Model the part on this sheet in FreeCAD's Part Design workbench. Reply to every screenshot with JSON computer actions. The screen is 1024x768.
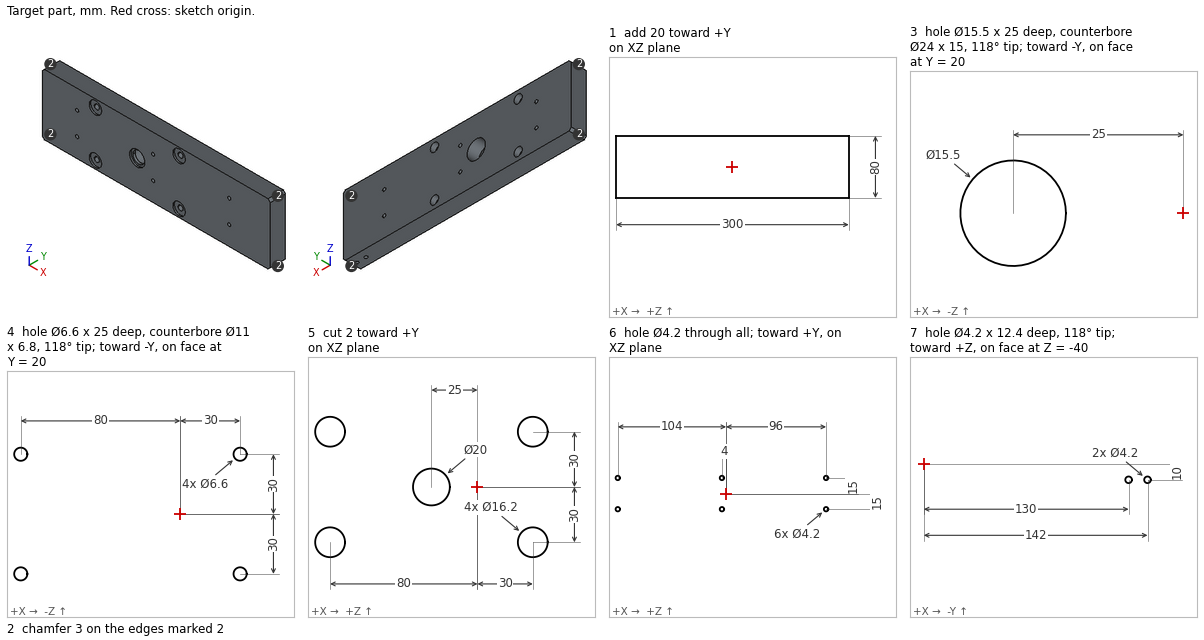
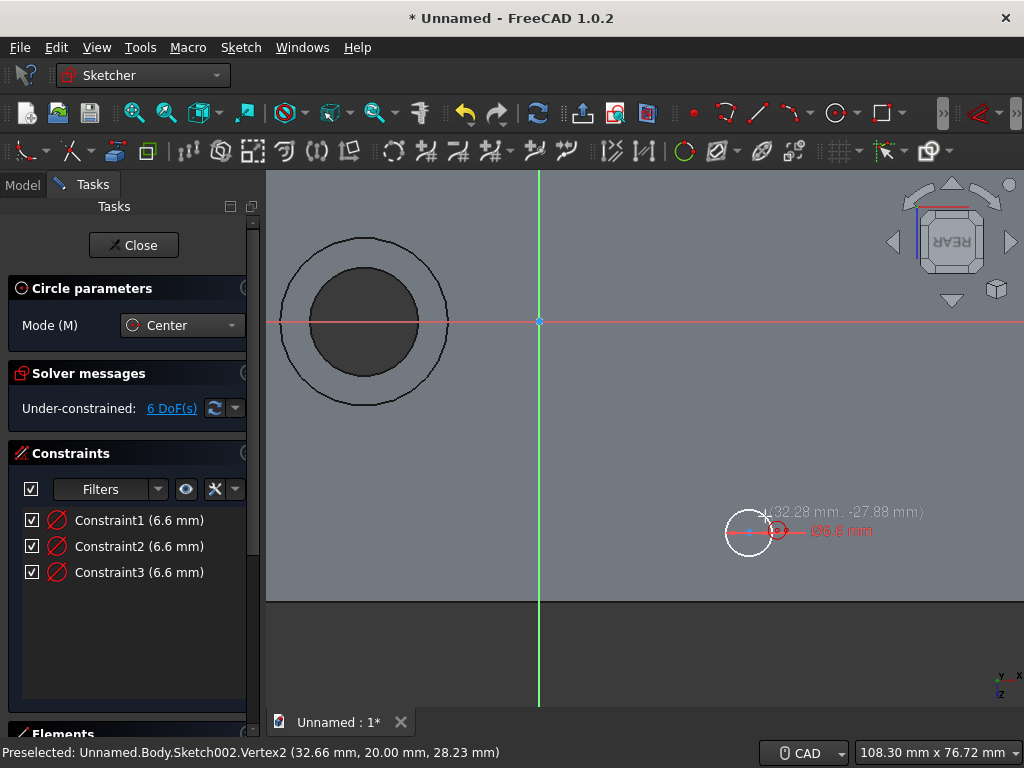
{"action": "scroll", "coordinate": [750, 534], "scroll_direction": "down", "scroll_amount": 4}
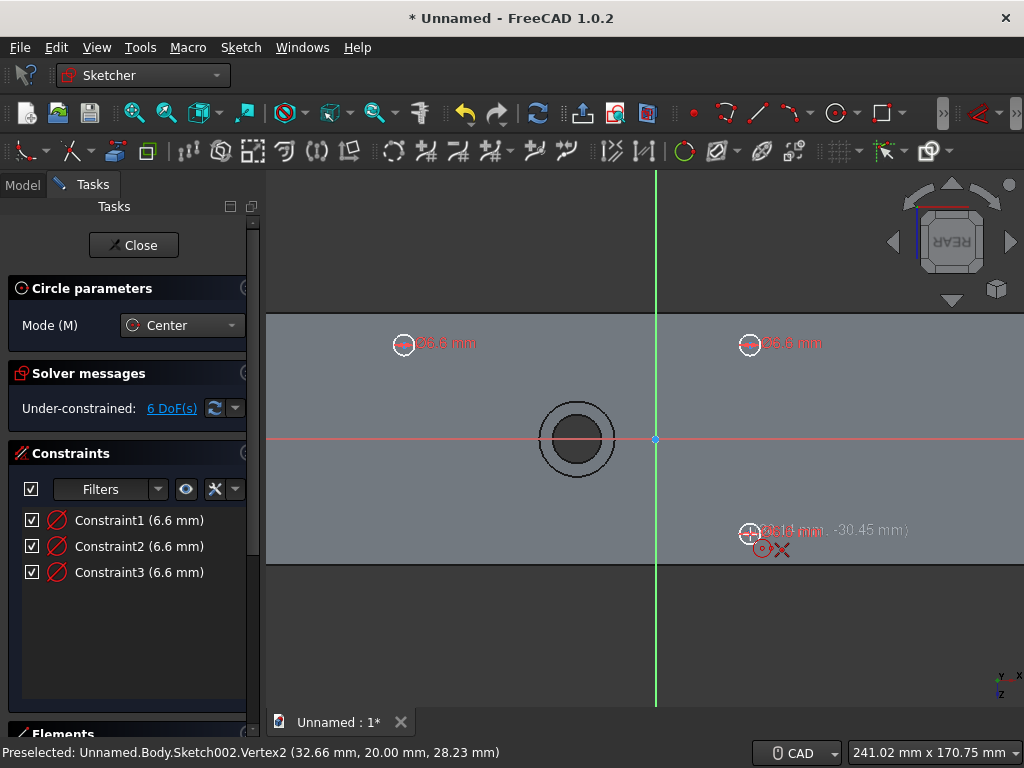
{"action": "scroll", "coordinate": [404, 533], "scroll_direction": "up", "scroll_amount": 4}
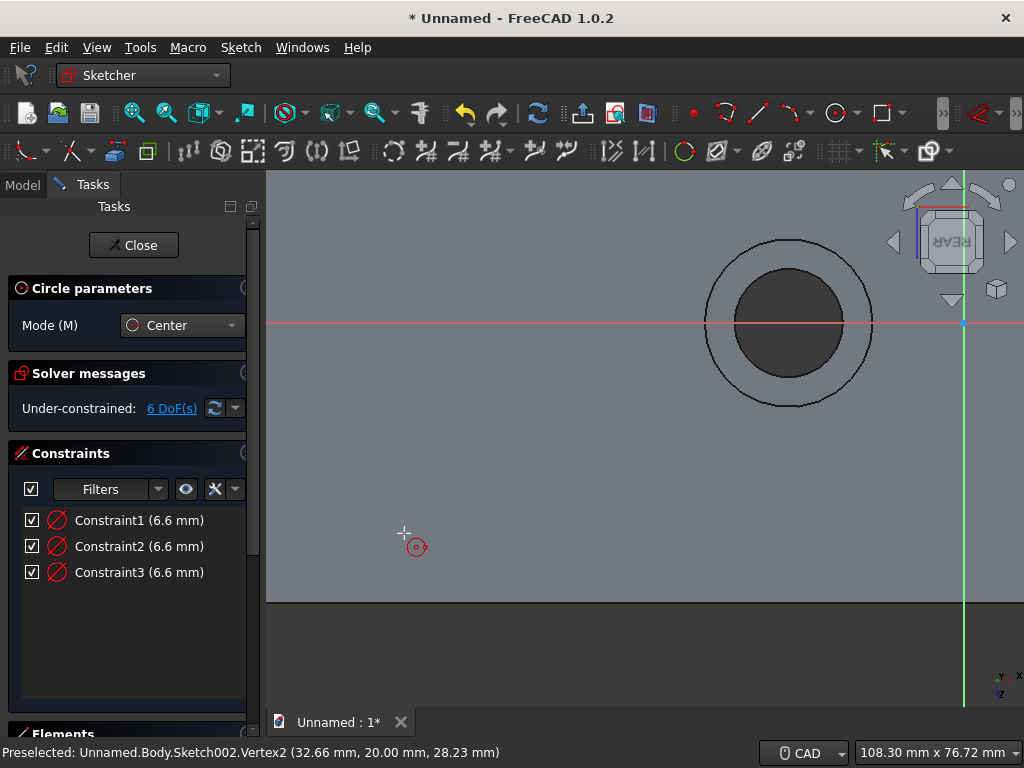
{"action": "left_click", "coordinate": [404, 533]}
{"action": "mouse_move", "coordinate": [420, 517]}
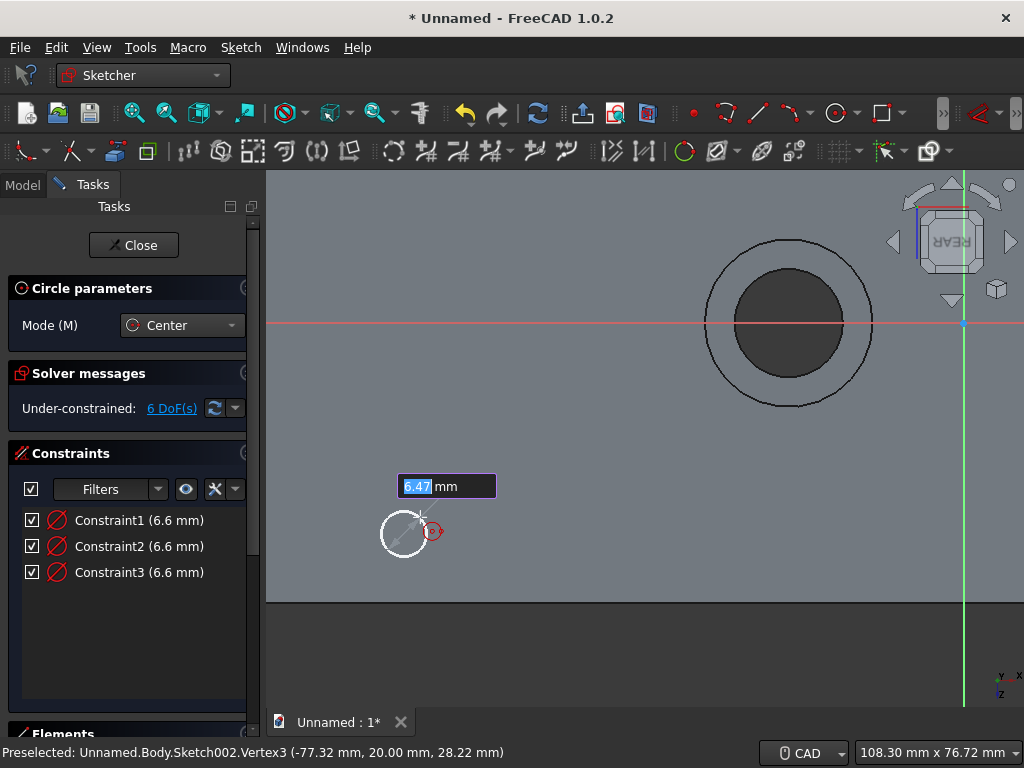
{"action": "type", "text": "6.6"}
{"action": "key", "text": "Return"}
{"action": "key", "text": "Escape"}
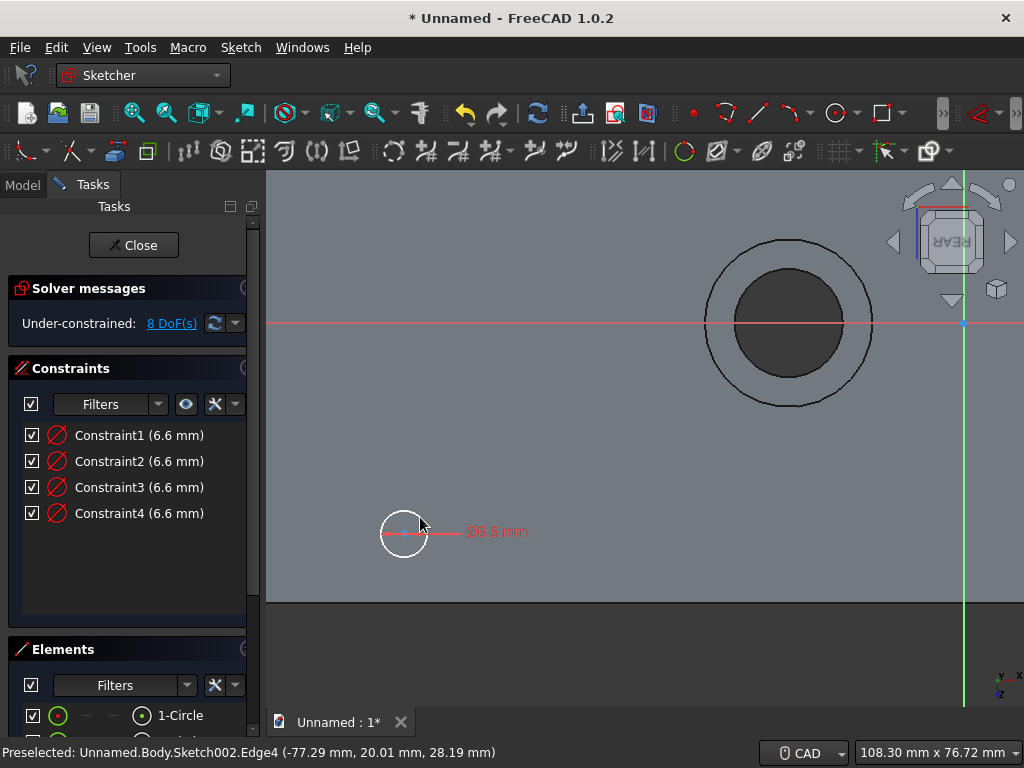
{"action": "scroll", "coordinate": [403, 533], "scroll_direction": "down", "scroll_amount": 4}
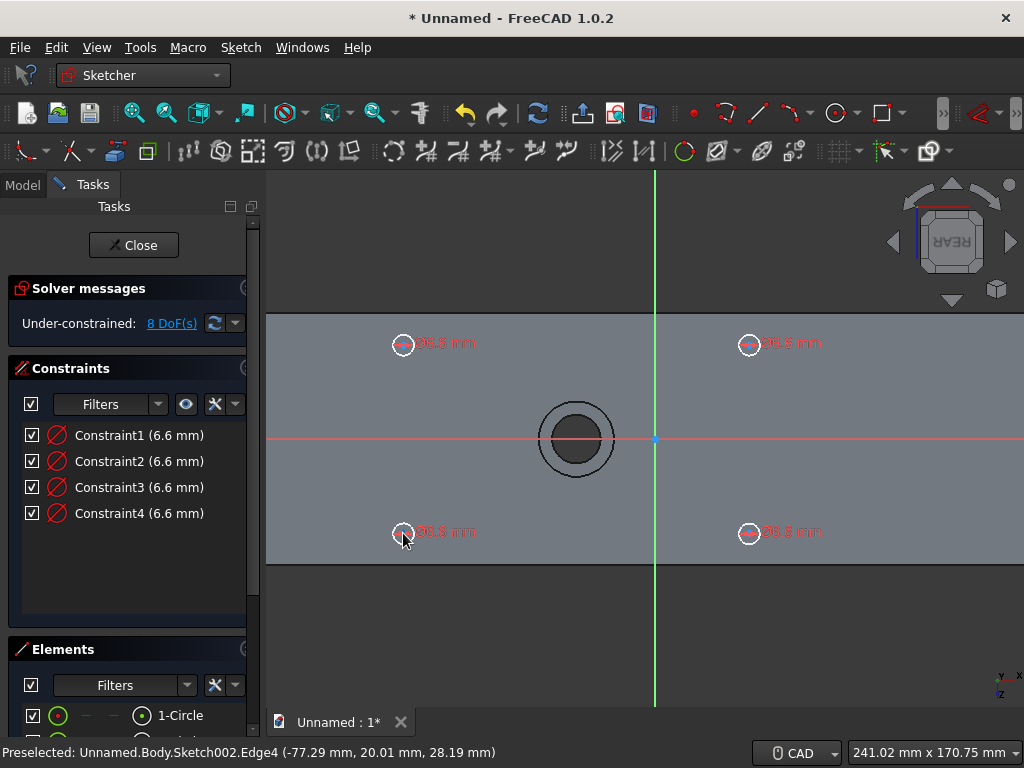
{"action": "left_click", "coordinate": [749, 345]}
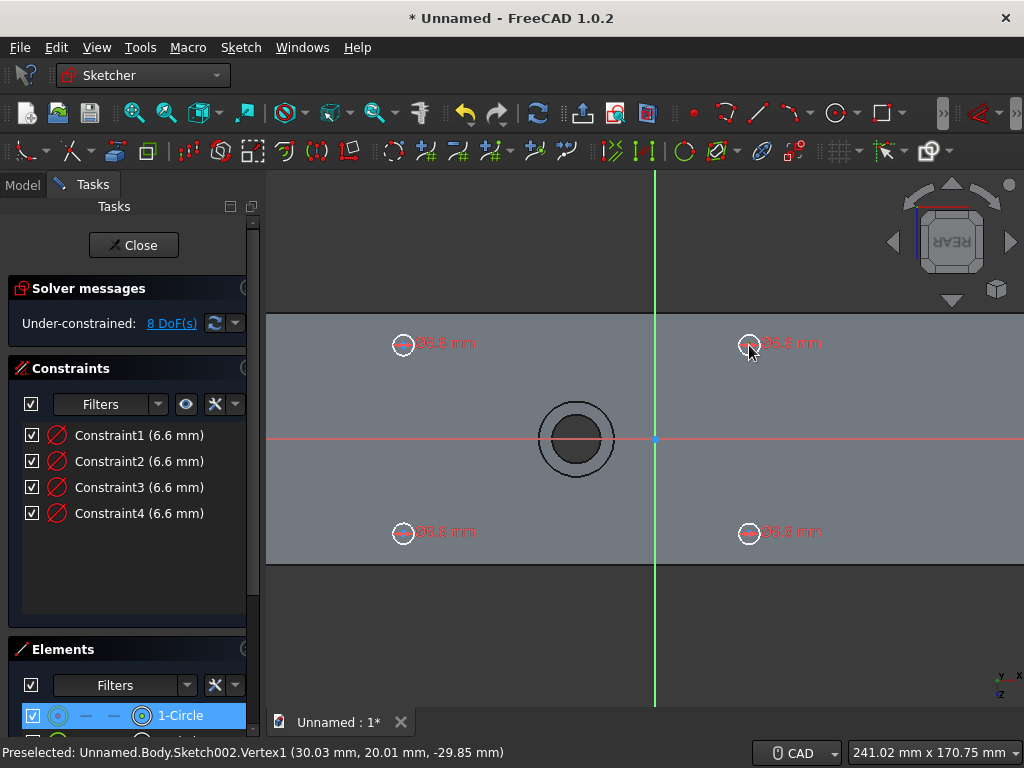
{"action": "left_click", "coordinate": [404, 345]}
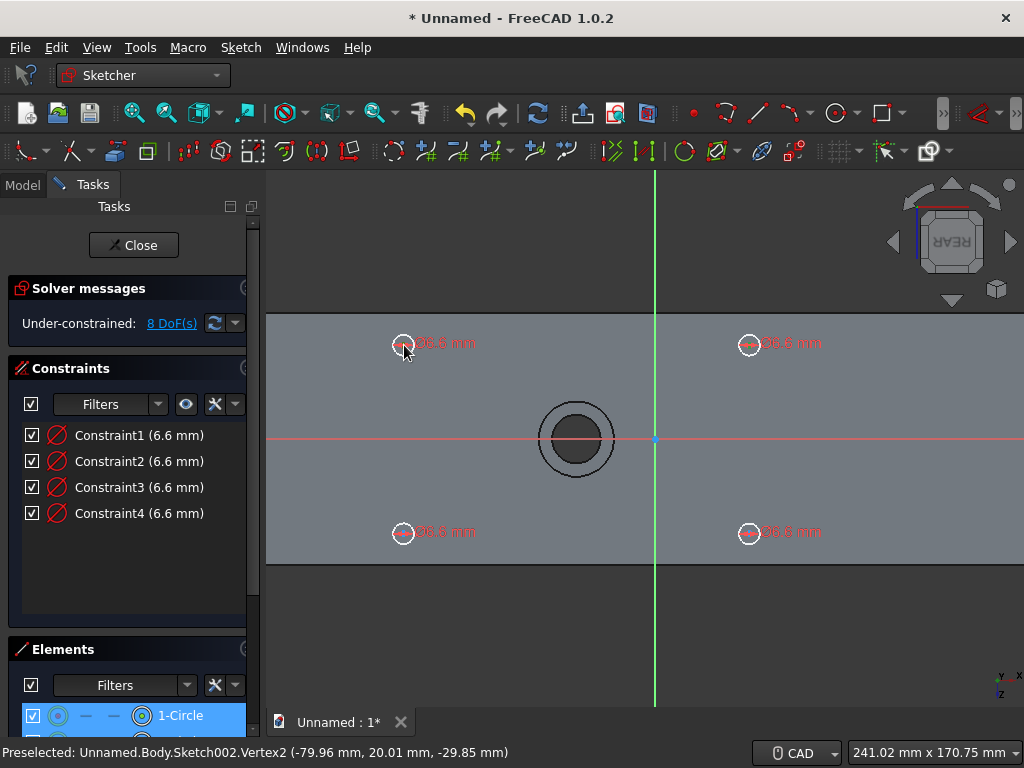
{"action": "key", "text": "h"}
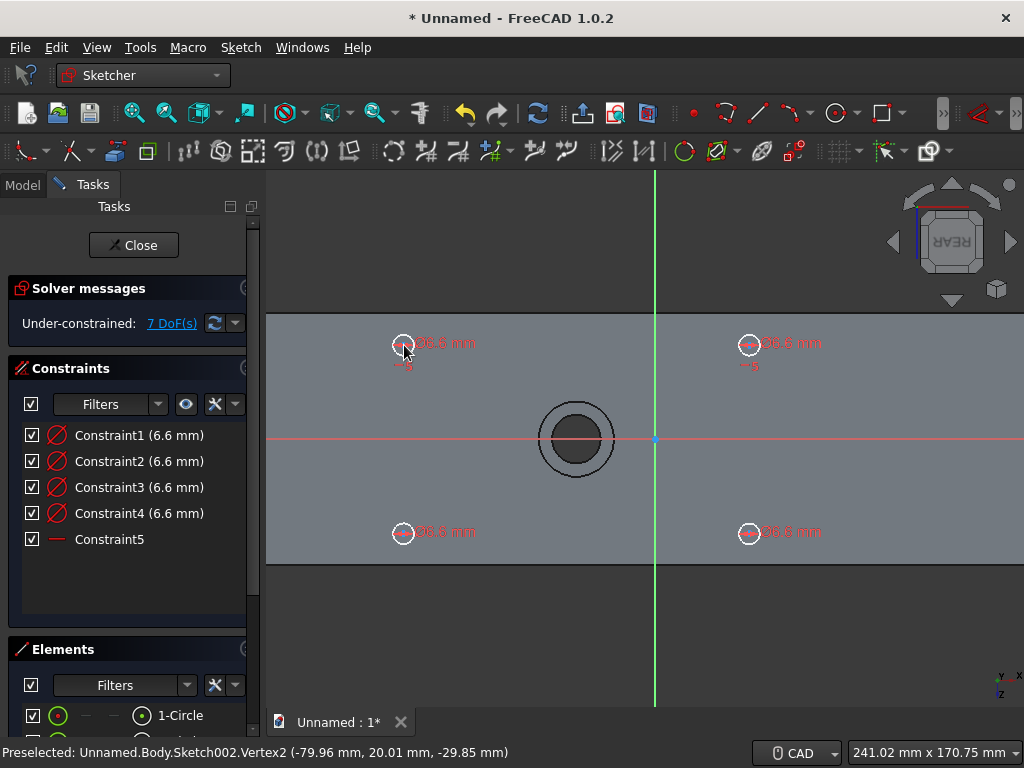
{"action": "left_click", "coordinate": [749, 345]}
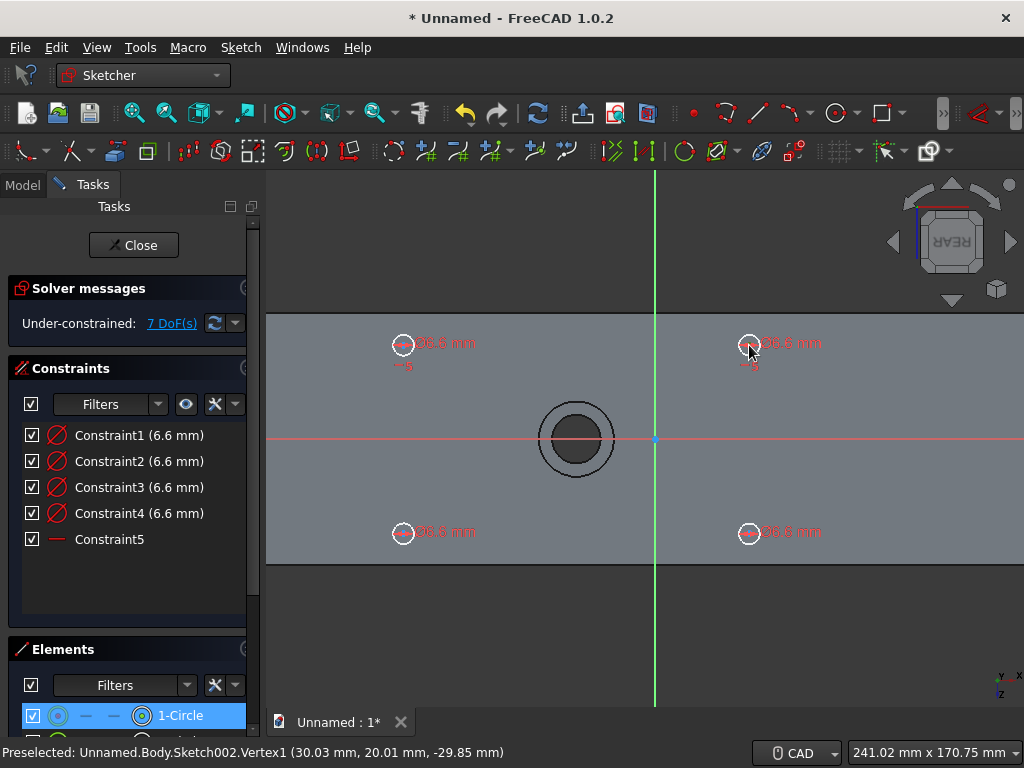
{"action": "left_click", "coordinate": [749, 534]}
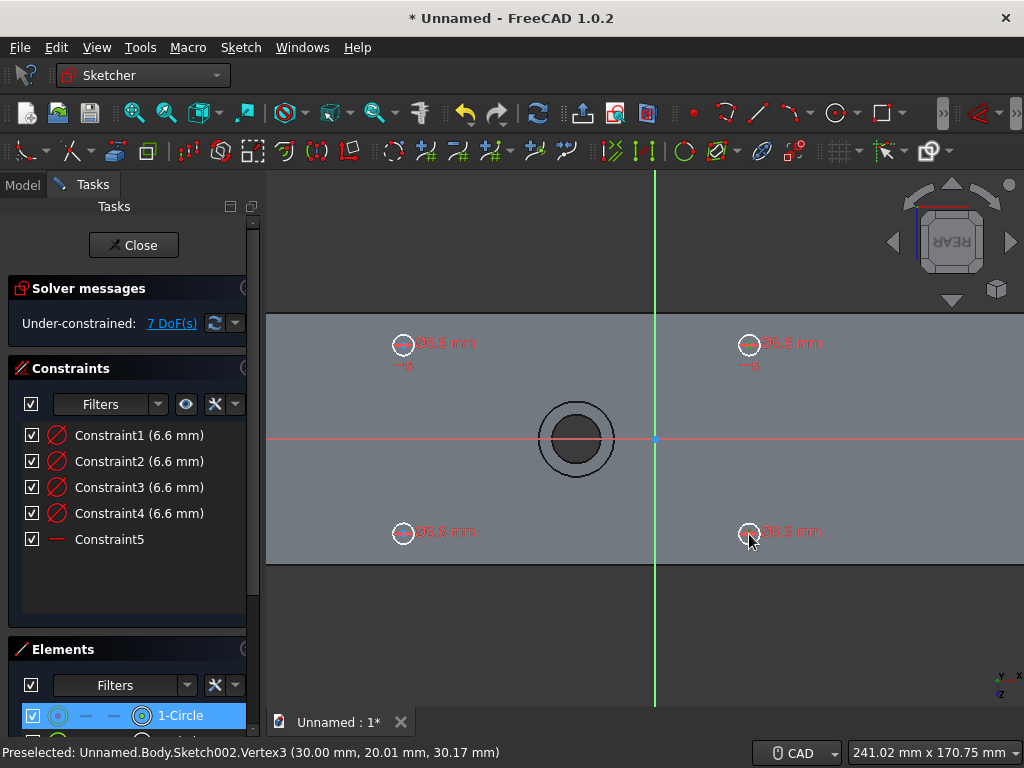
{"action": "key", "text": "v"}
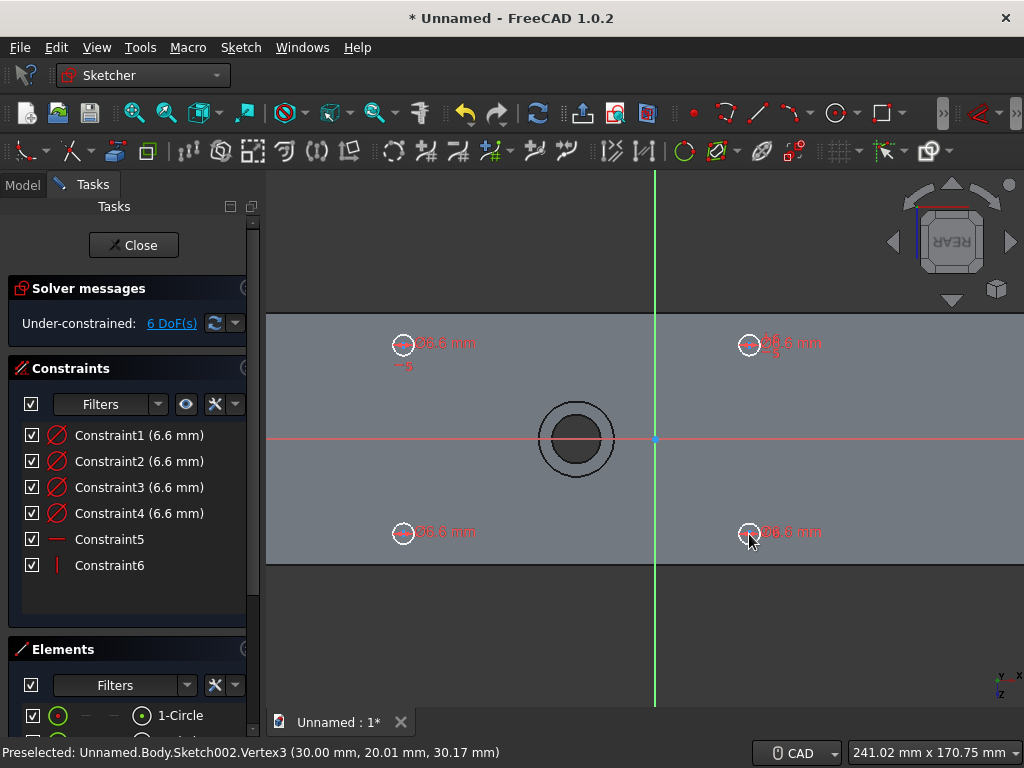
{"action": "left_click", "coordinate": [404, 345]}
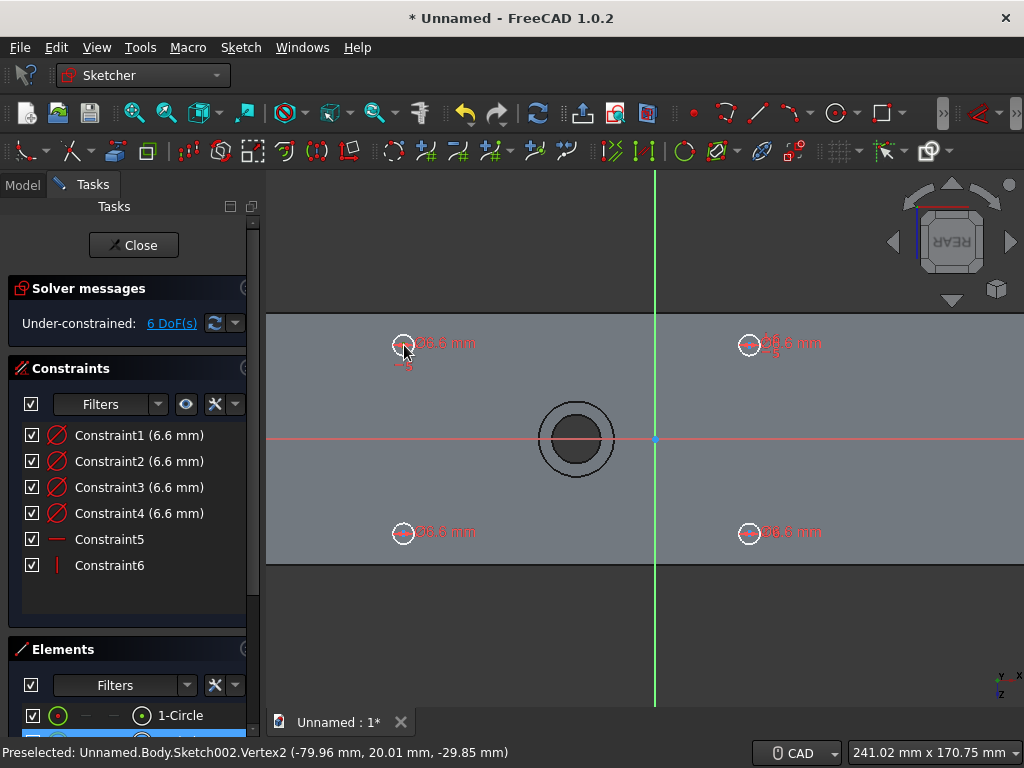
{"action": "left_click", "coordinate": [404, 534]}